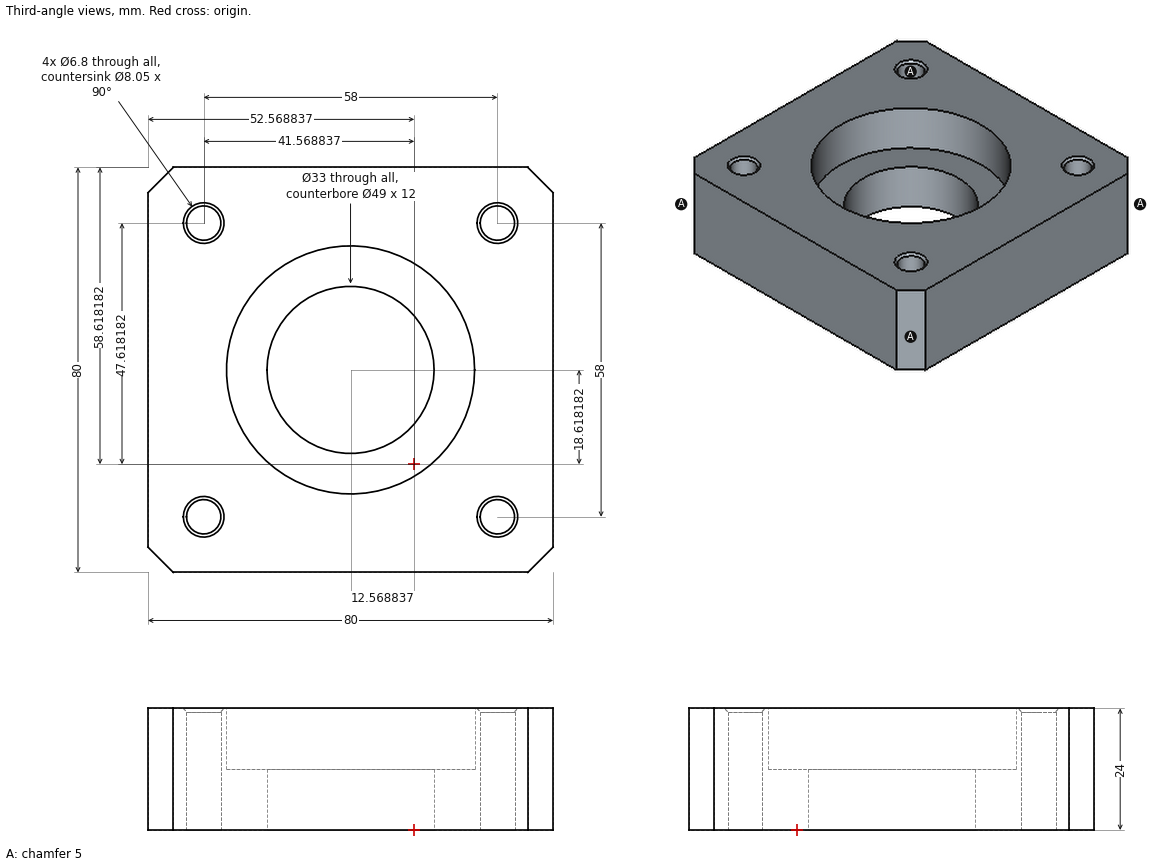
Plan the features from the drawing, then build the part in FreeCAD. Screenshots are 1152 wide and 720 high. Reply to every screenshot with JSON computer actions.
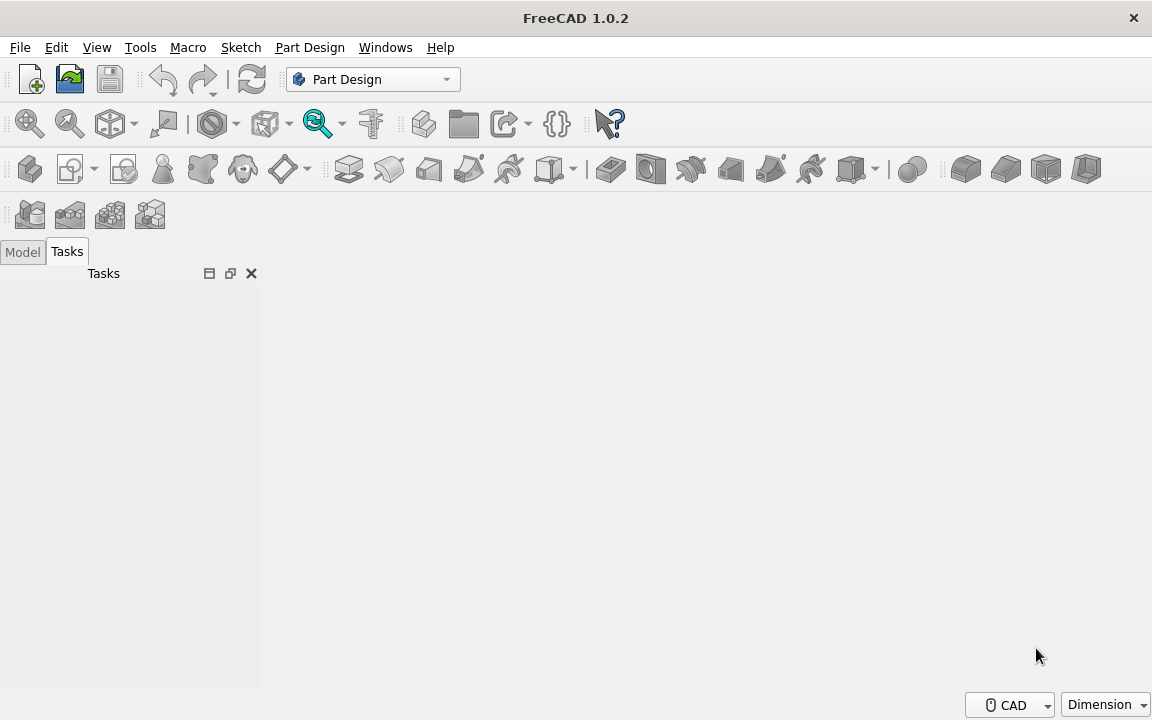
{"action": "left_click", "coordinate": [30, 80]}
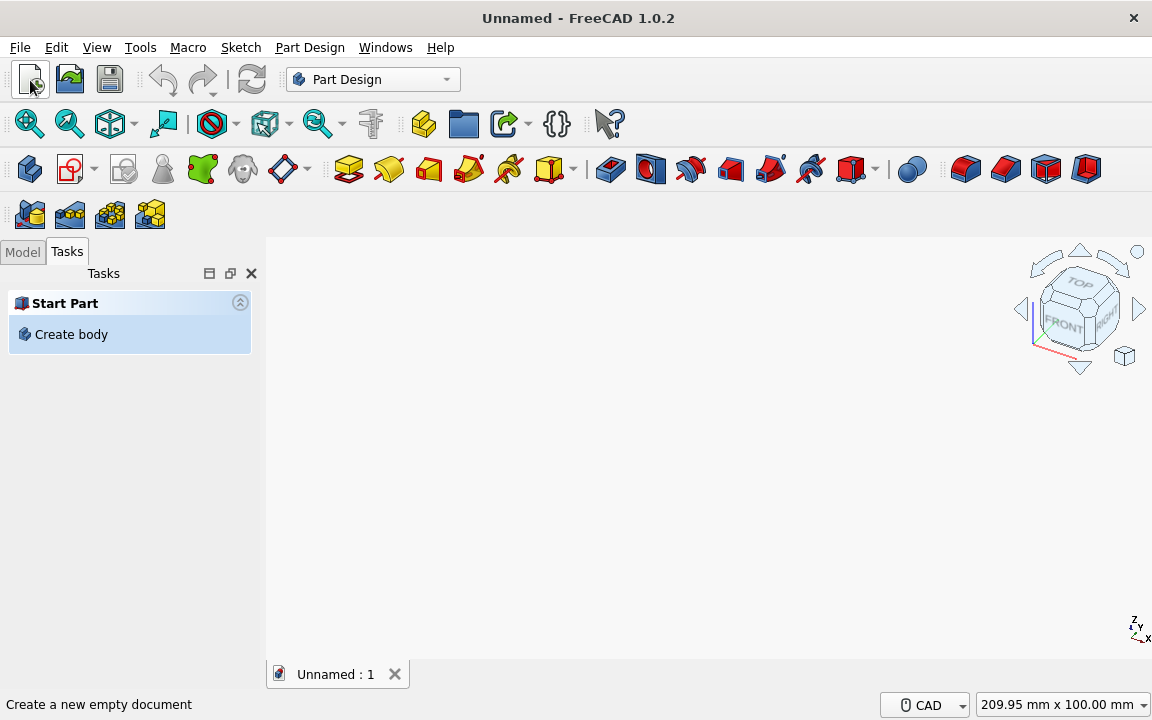
{"action": "left_click", "coordinate": [70, 170]}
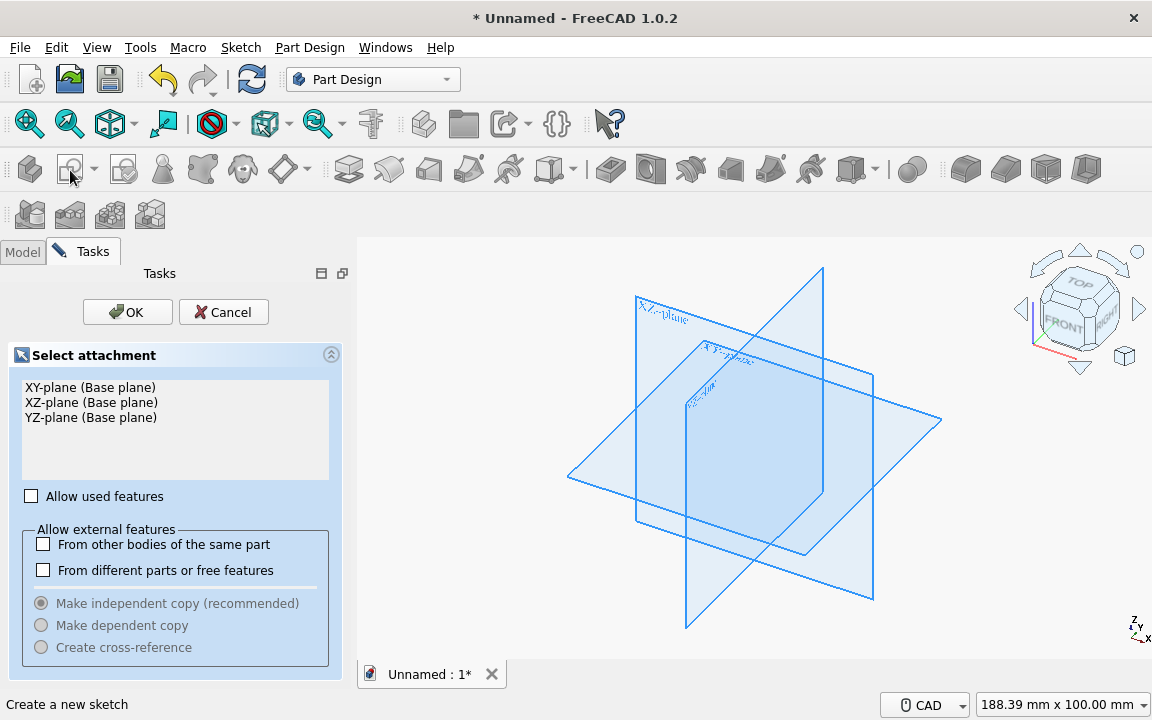
{"action": "left_click", "coordinate": [82, 388]}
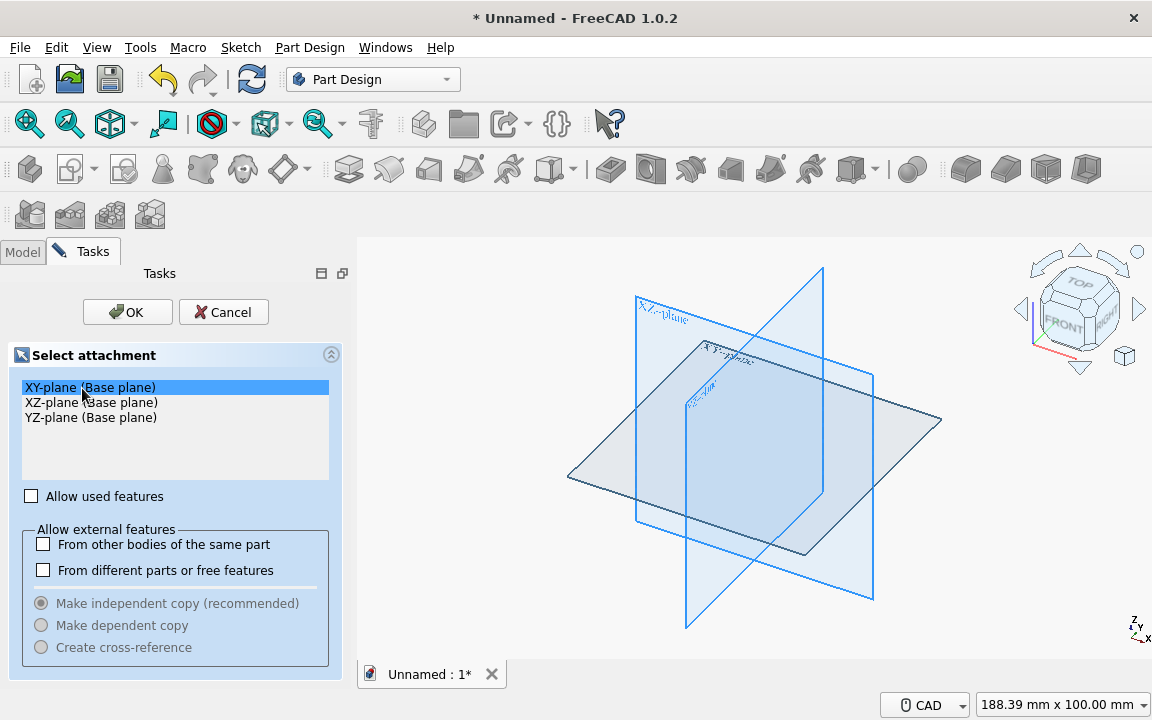
{"action": "left_click", "coordinate": [128, 312]}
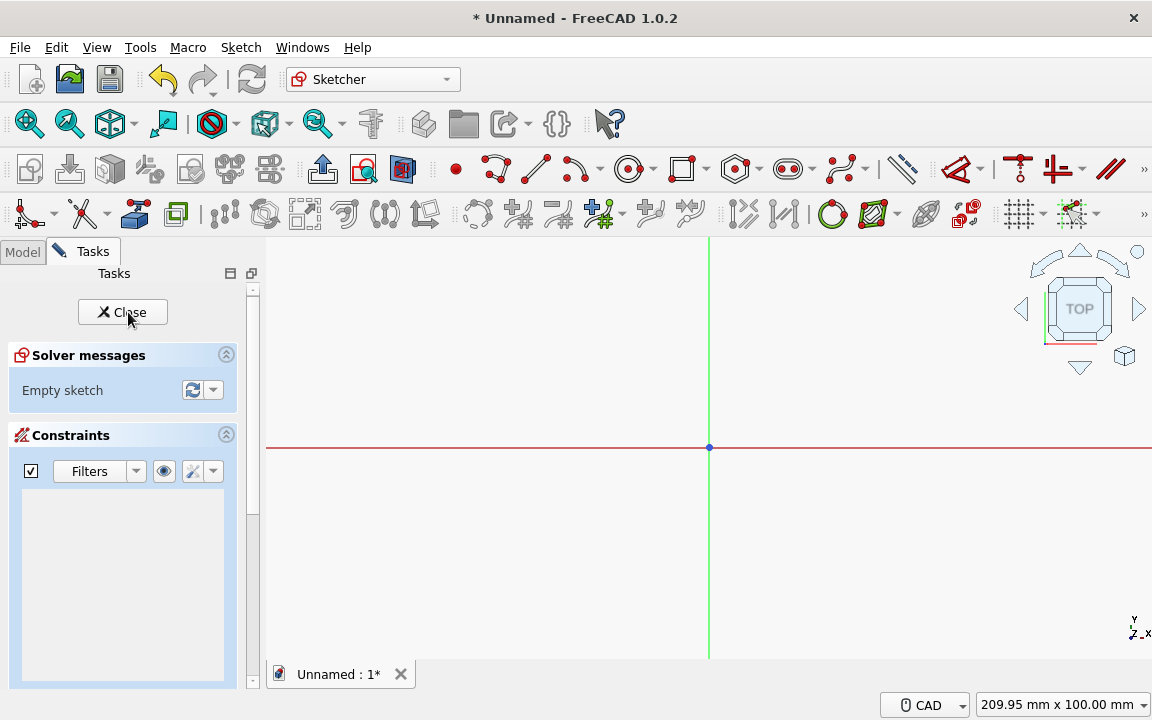
{"action": "scroll", "coordinate": [609, 608], "scroll_direction": "down", "scroll_amount": 2}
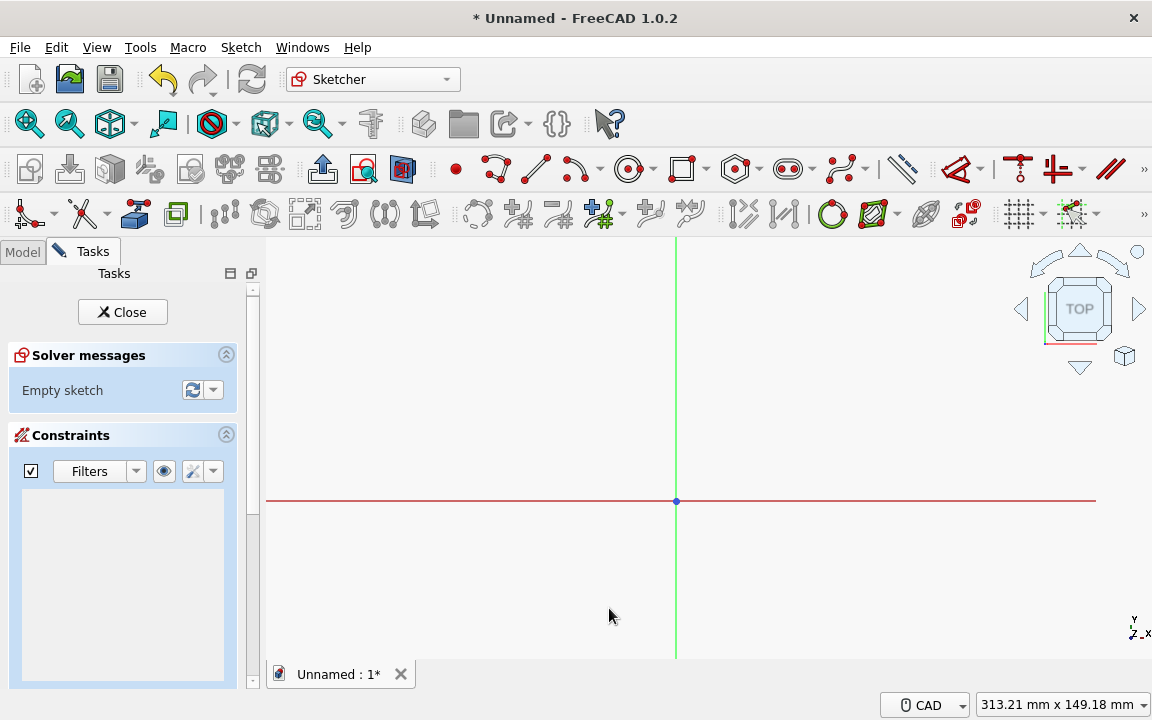
{"action": "left_click", "coordinate": [682, 170]}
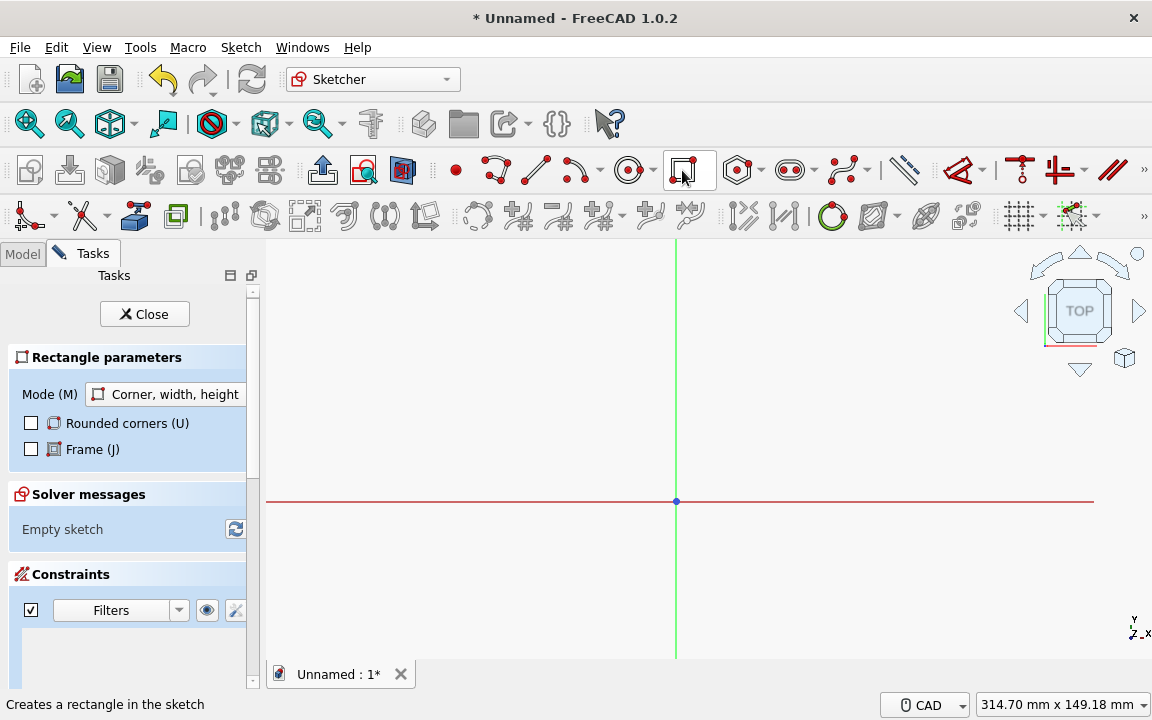
{"action": "left_click", "coordinate": [528, 337]}
{"action": "left_click", "coordinate": [754, 562]}
{"action": "key", "text": "Escape"}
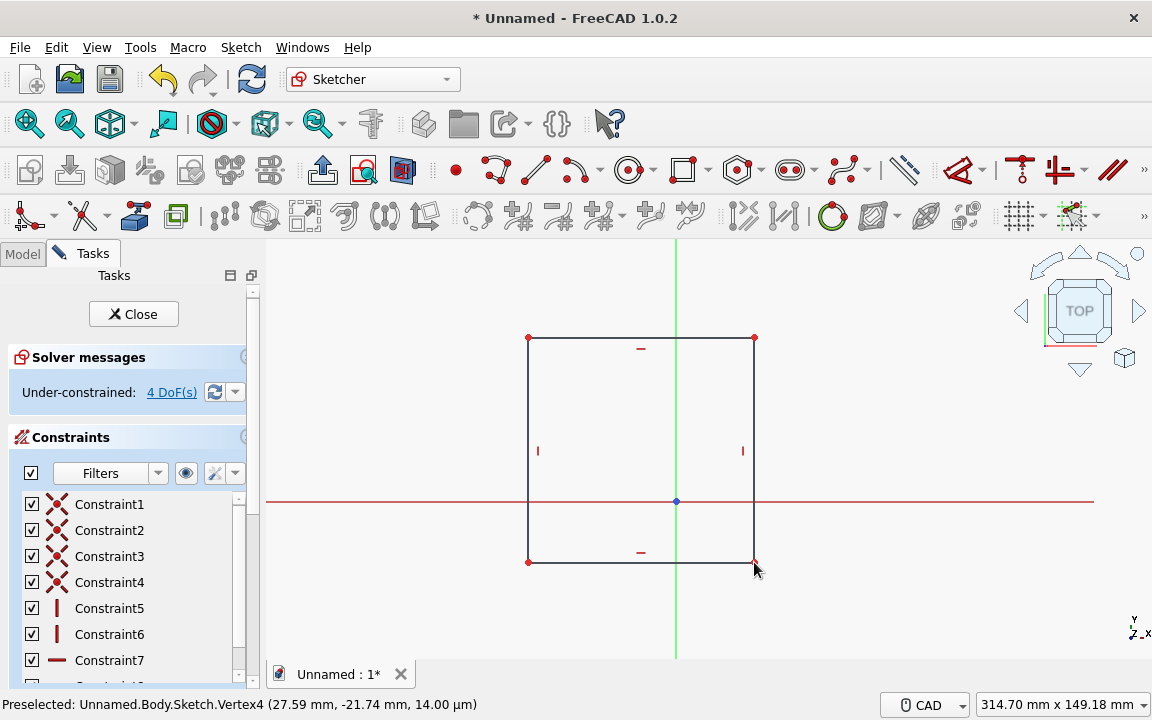
{"action": "left_click", "coordinate": [528, 405]}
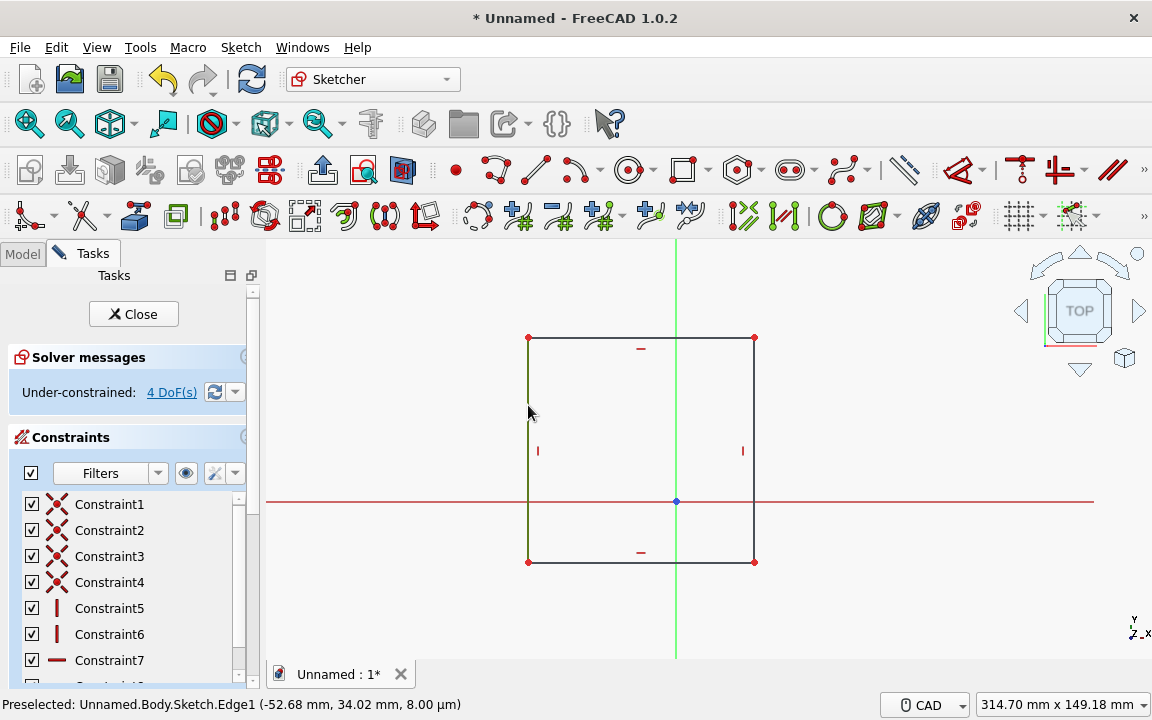
{"action": "left_click", "coordinate": [984, 170]}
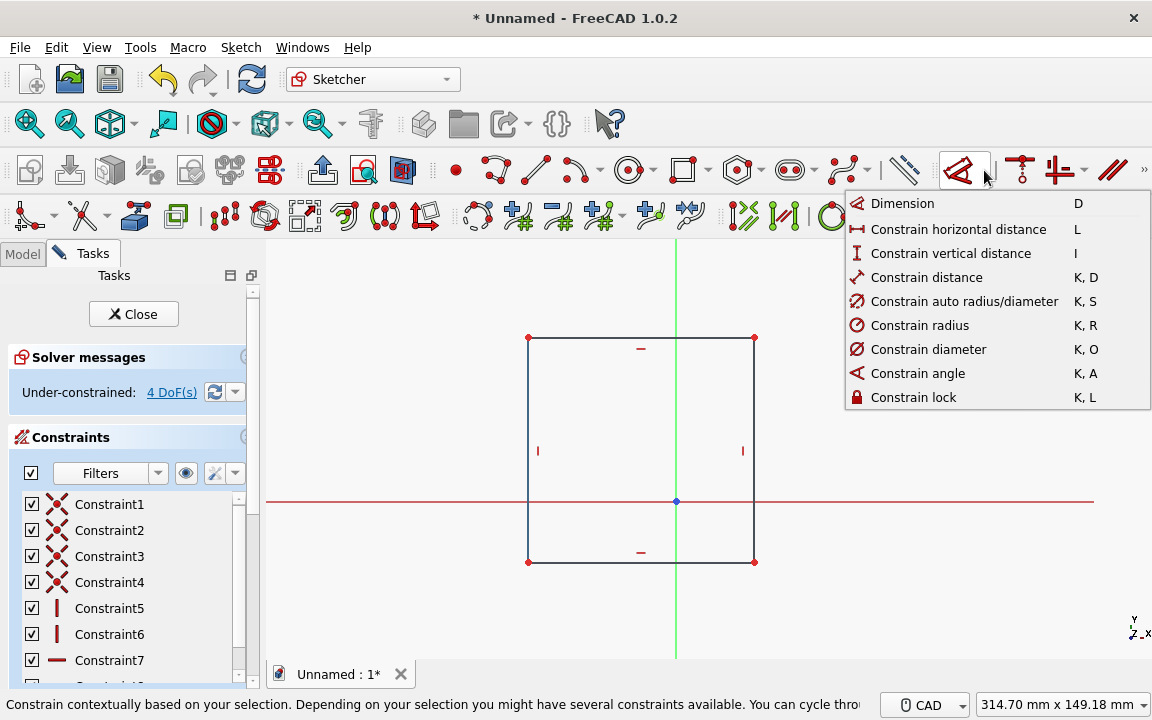
{"action": "left_click", "coordinate": [998, 253]}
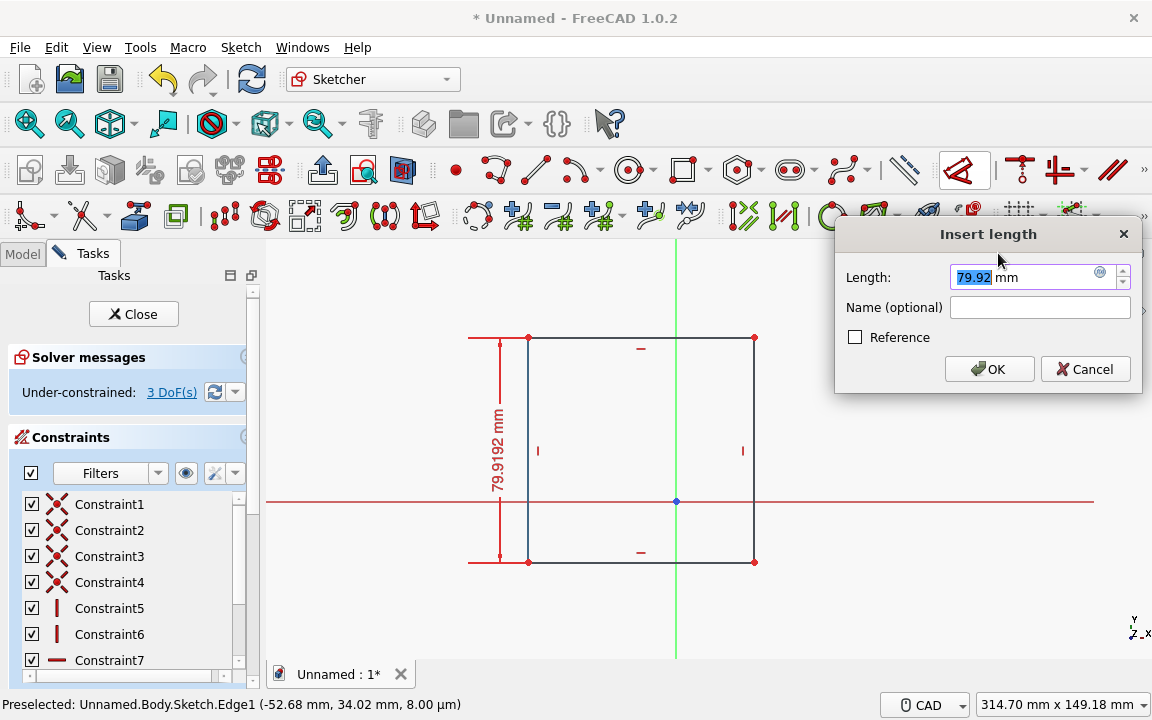
{"action": "type", "text": "80"}
{"action": "key", "text": "Return"}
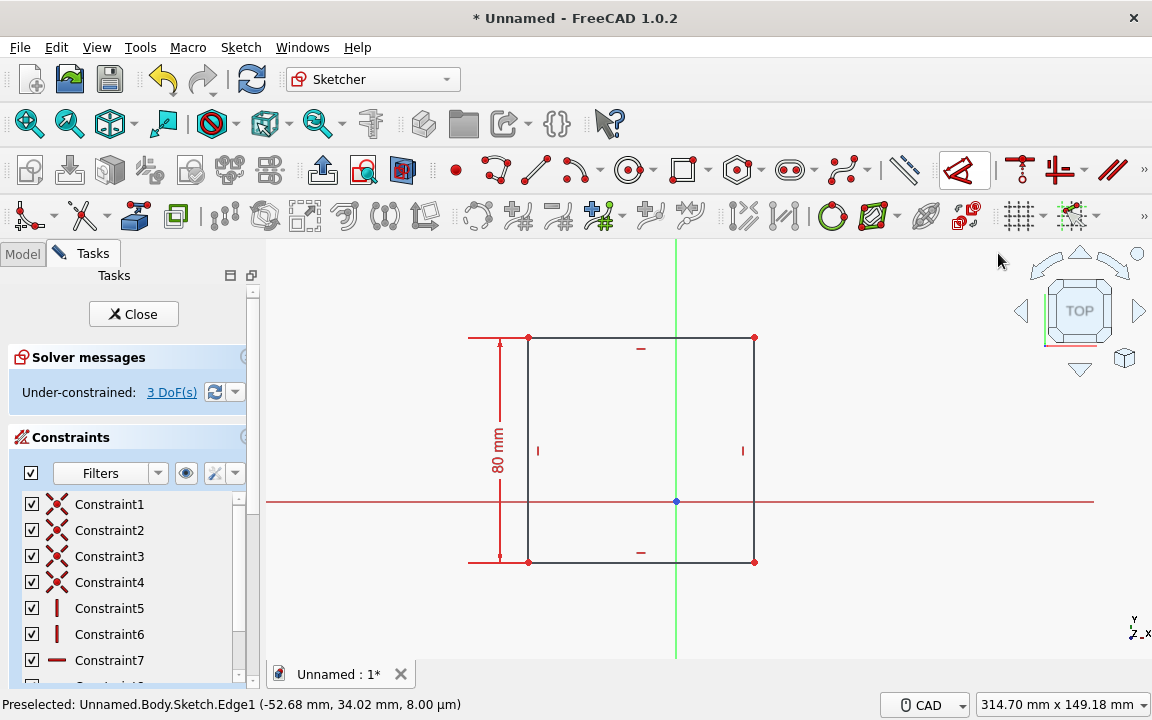
{"action": "left_click", "coordinate": [596, 563]}